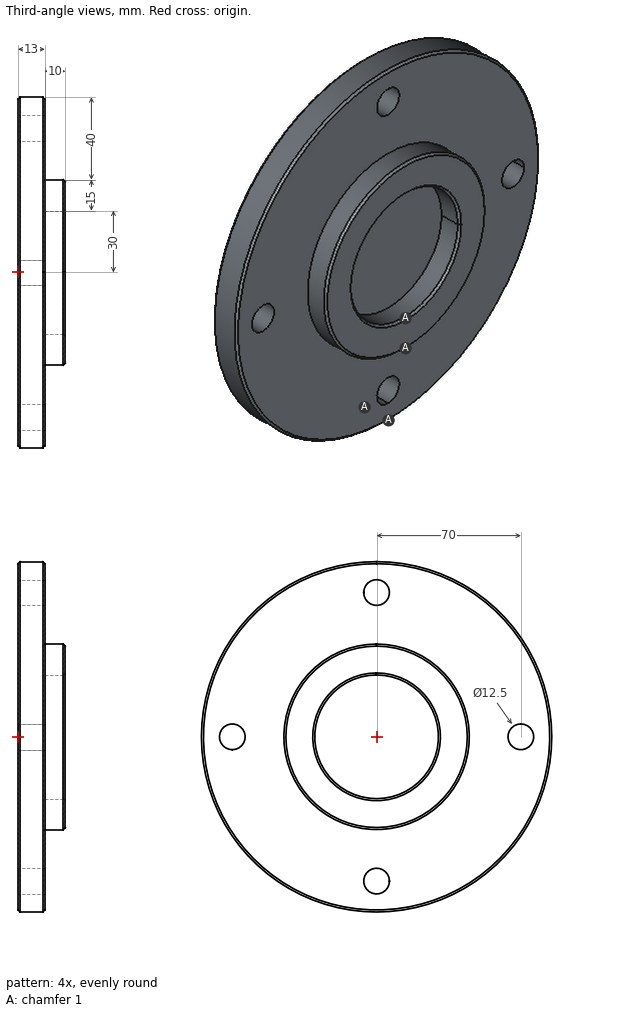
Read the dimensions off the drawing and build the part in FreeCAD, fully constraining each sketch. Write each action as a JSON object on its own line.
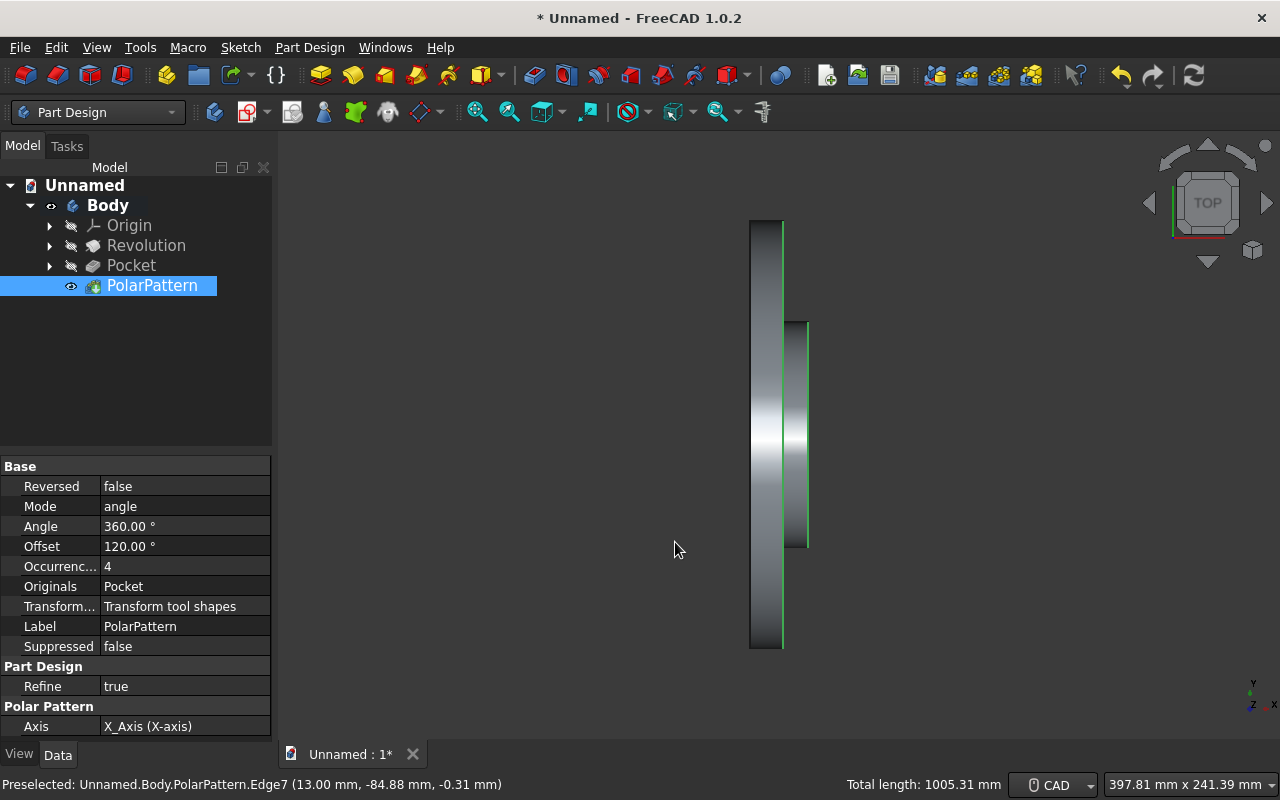
{"action": "left_click", "coordinate": [750, 607], "text": "ctrl"}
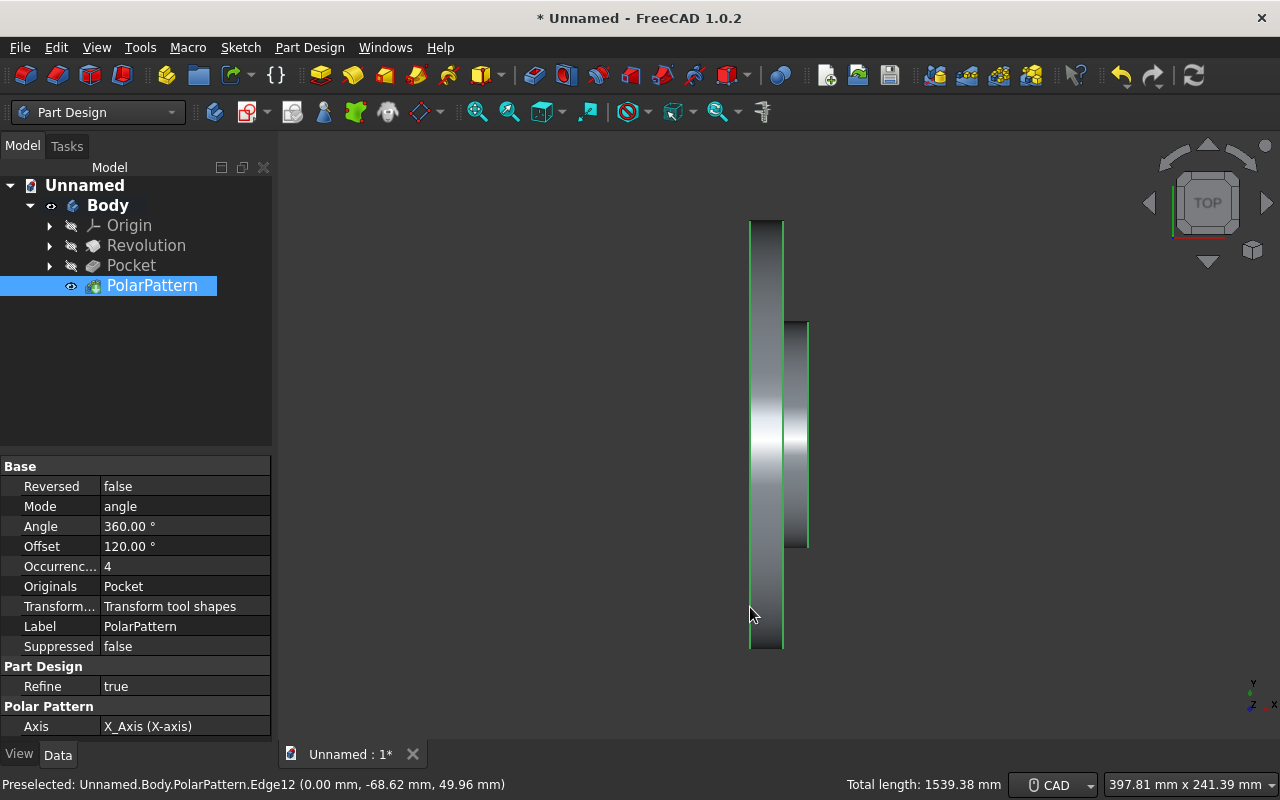
{"action": "left_click", "coordinate": [58, 76]}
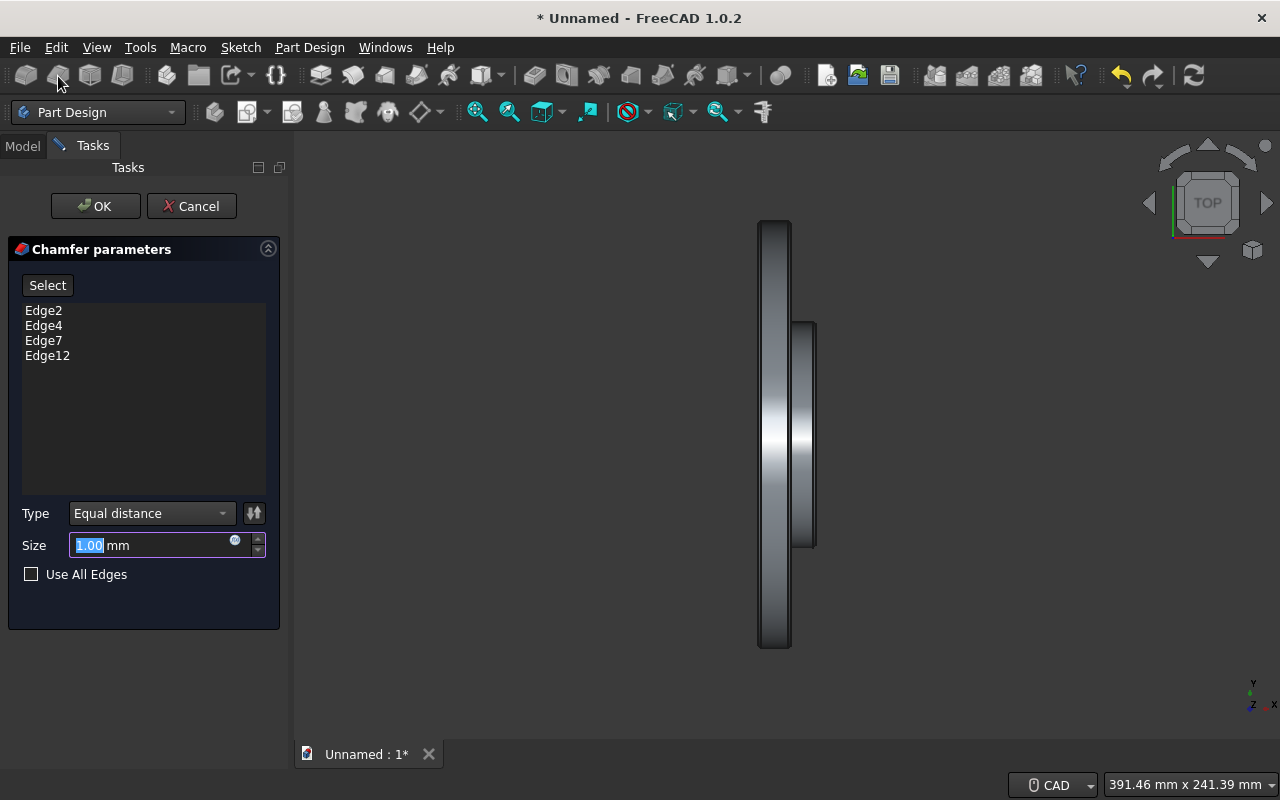
{"action": "type", "text": "1"}
{"action": "key", "text": "Tab"}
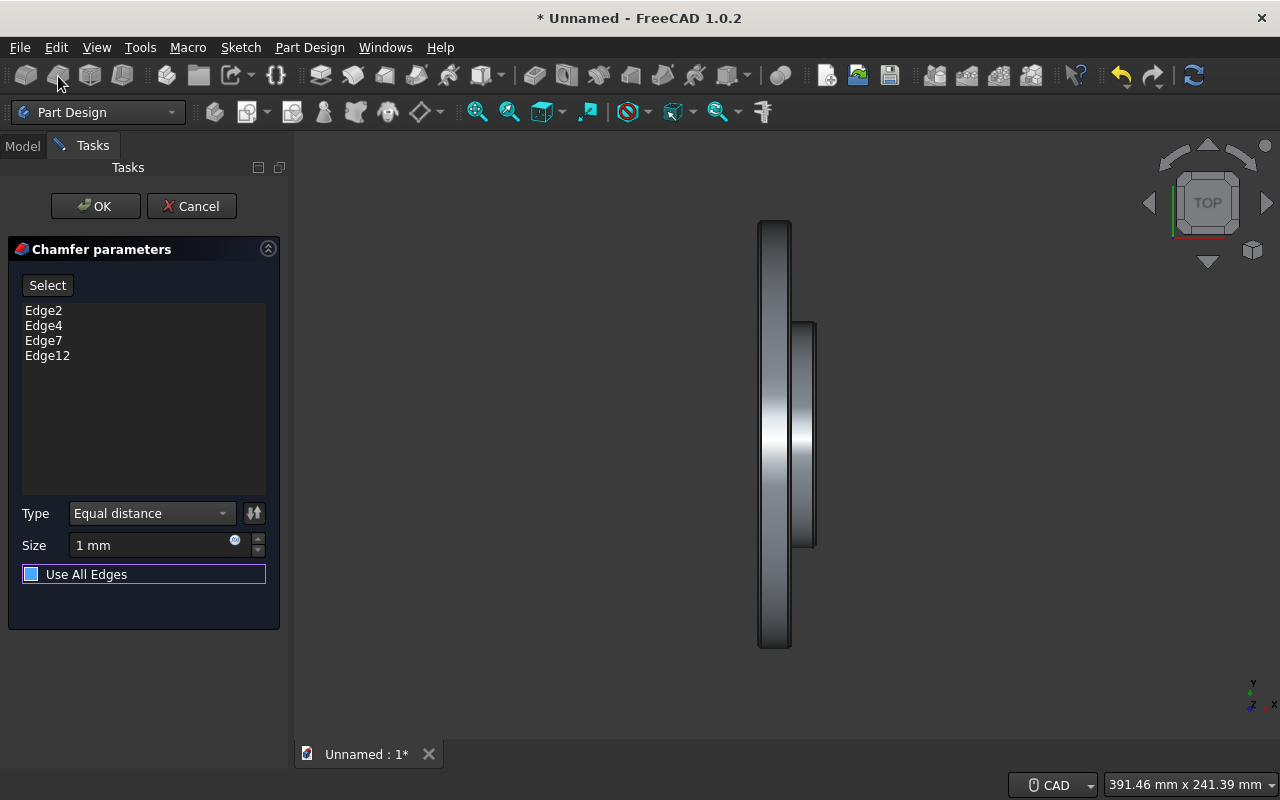
{"action": "left_click", "coordinate": [96, 206]}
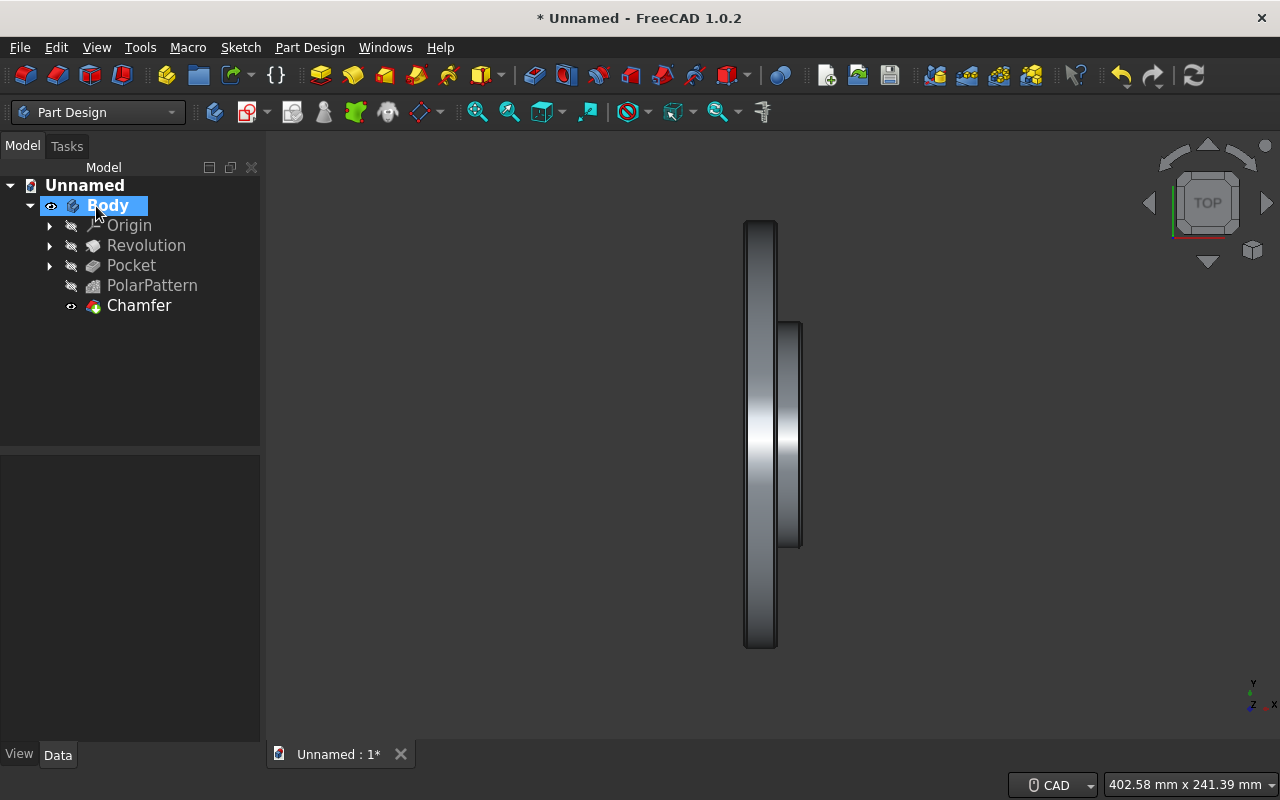
{"action": "key", "text": "0"}